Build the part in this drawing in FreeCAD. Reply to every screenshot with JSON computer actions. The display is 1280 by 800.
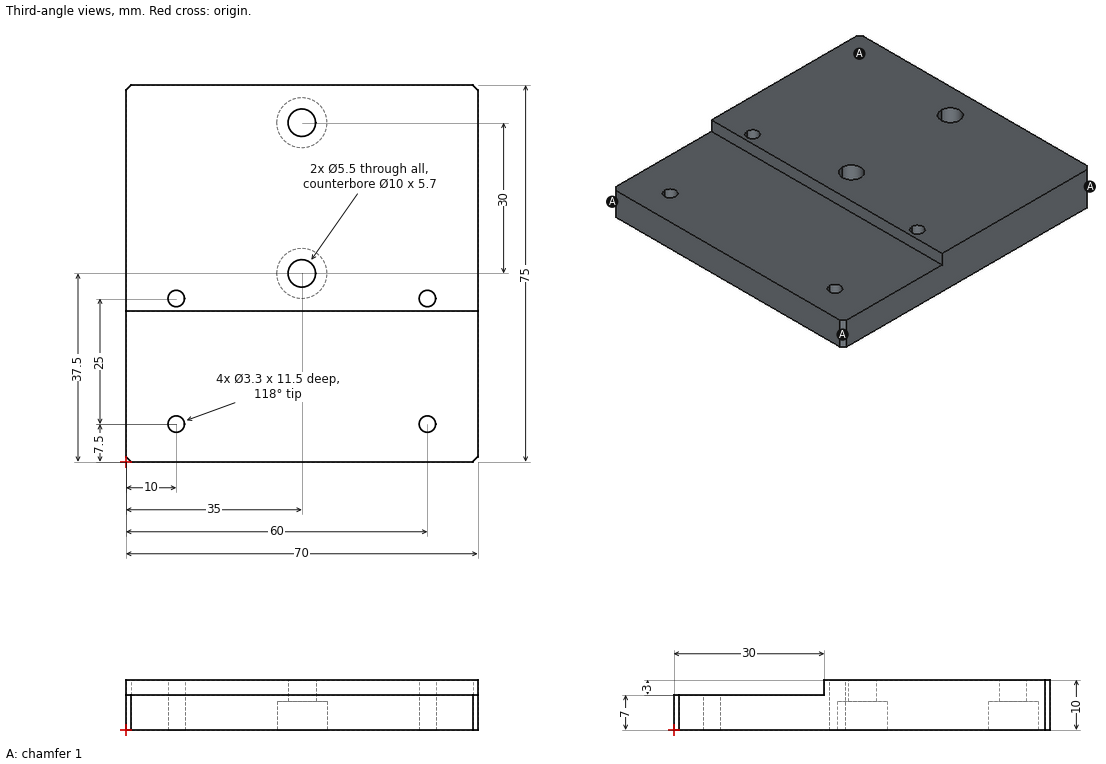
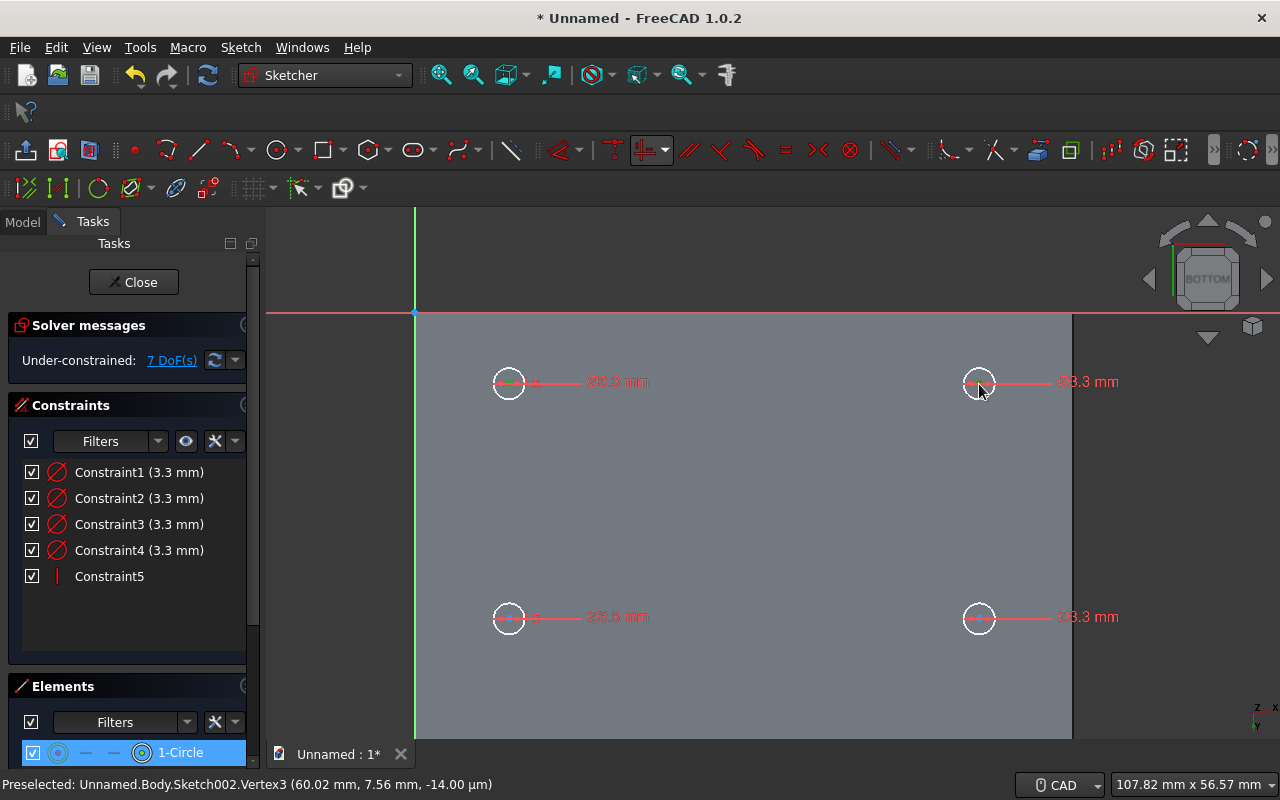
{"action": "key", "text": "h"}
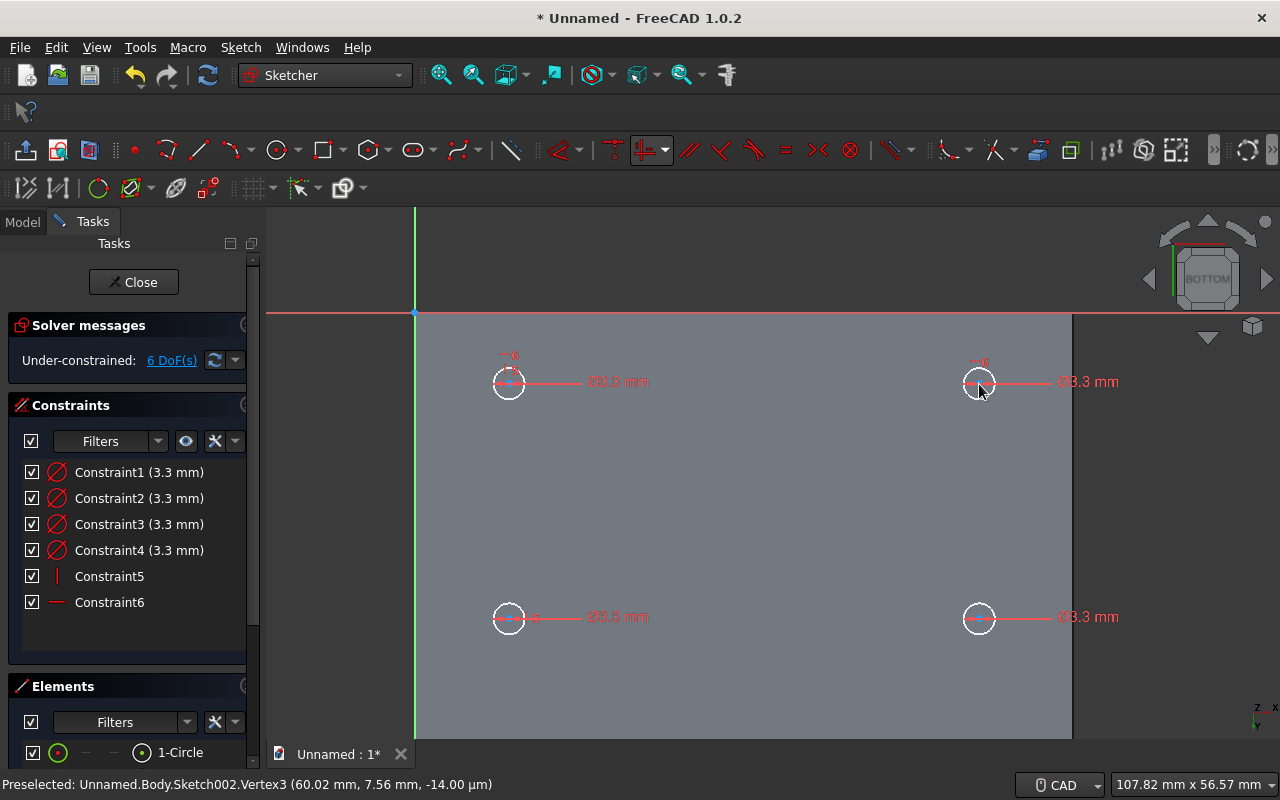
{"action": "left_click", "coordinate": [979, 384]}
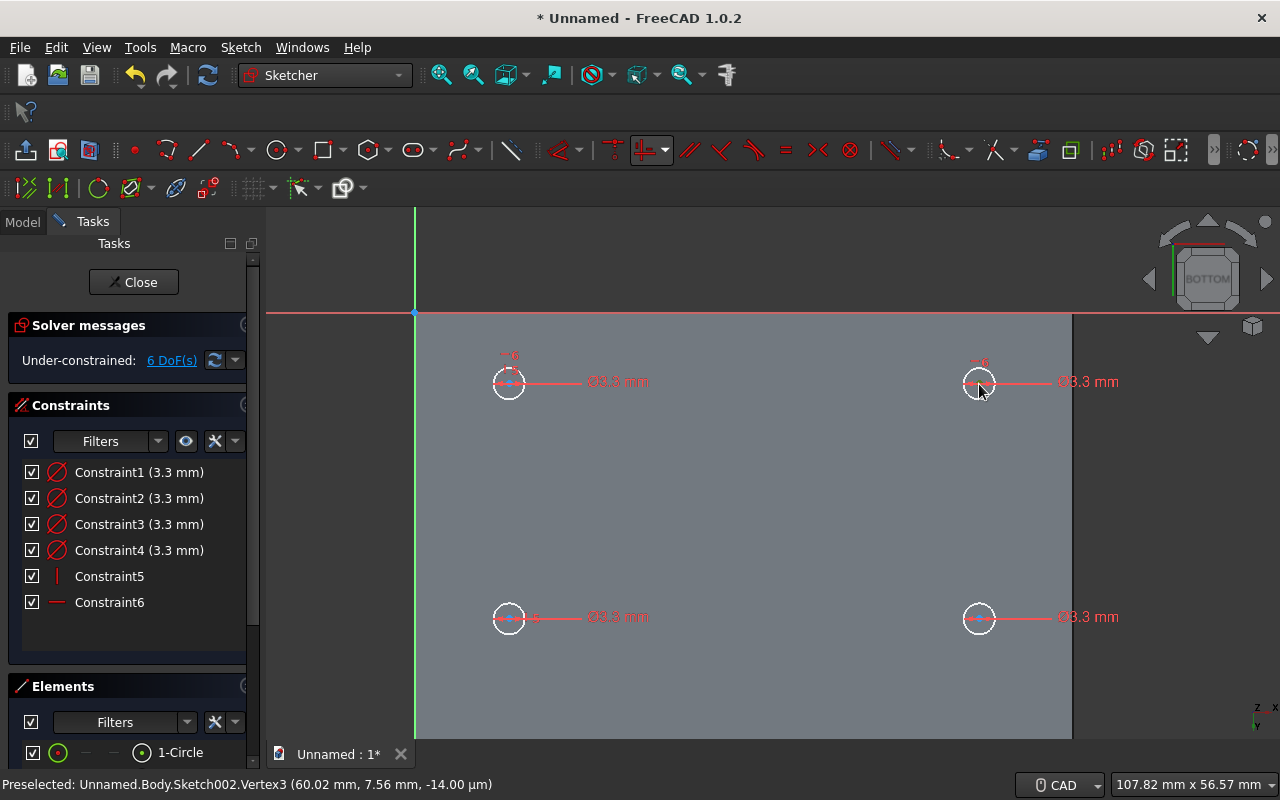
{"action": "left_click", "coordinate": [979, 619]}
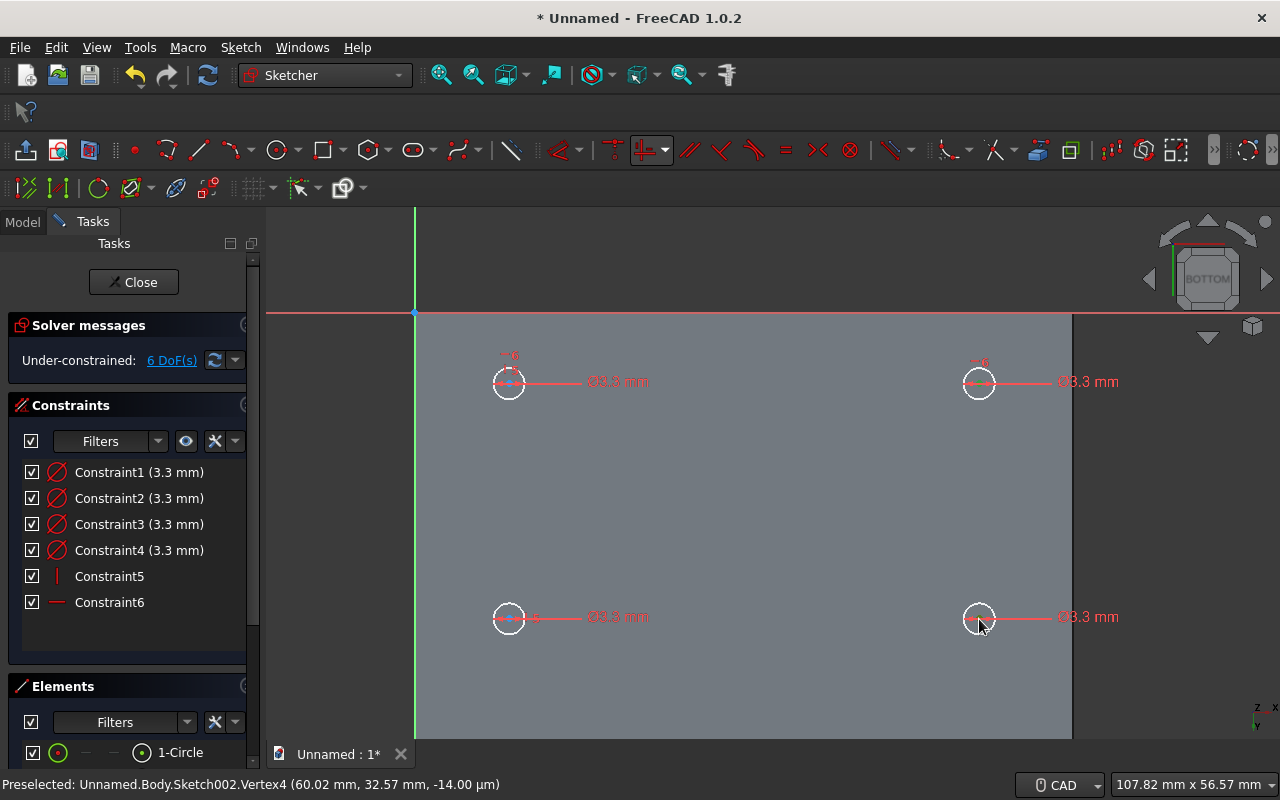
{"action": "key", "text": "v"}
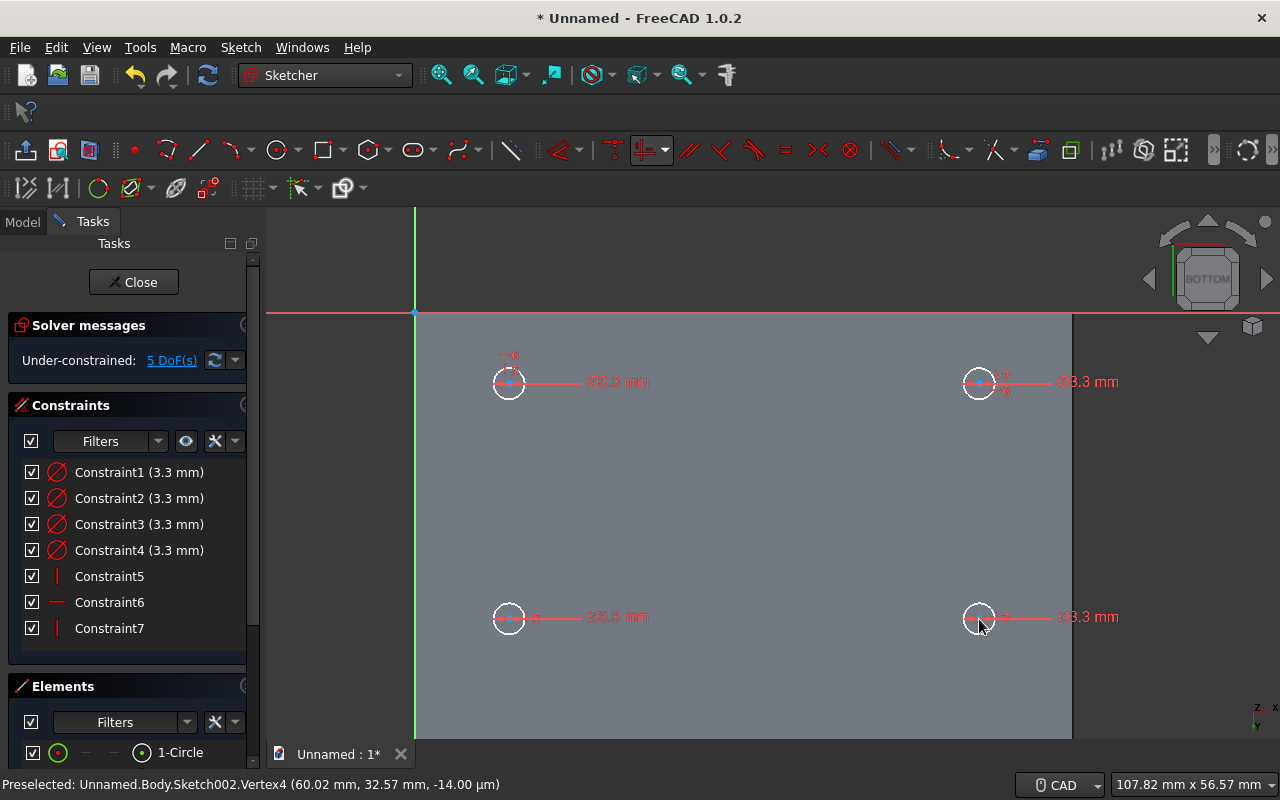
{"action": "left_click", "coordinate": [509, 619]}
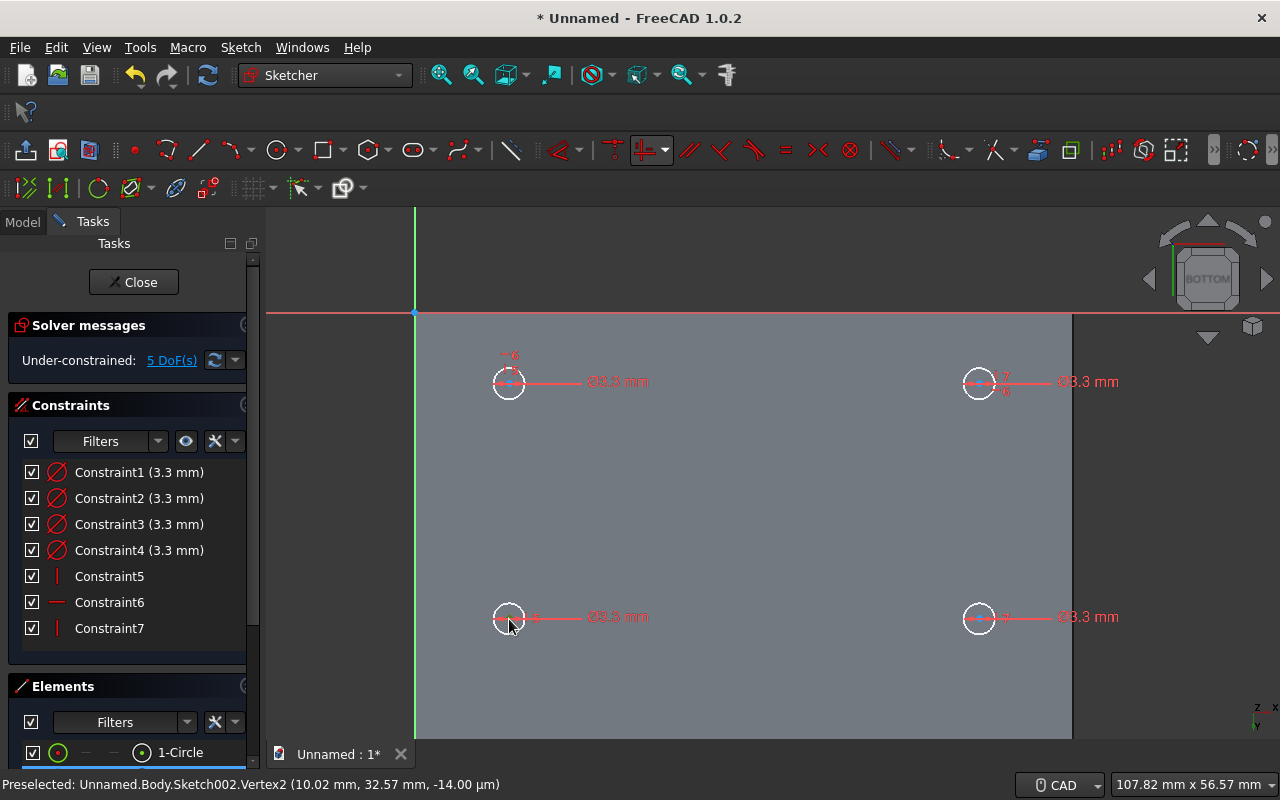
{"action": "left_click", "coordinate": [979, 619]}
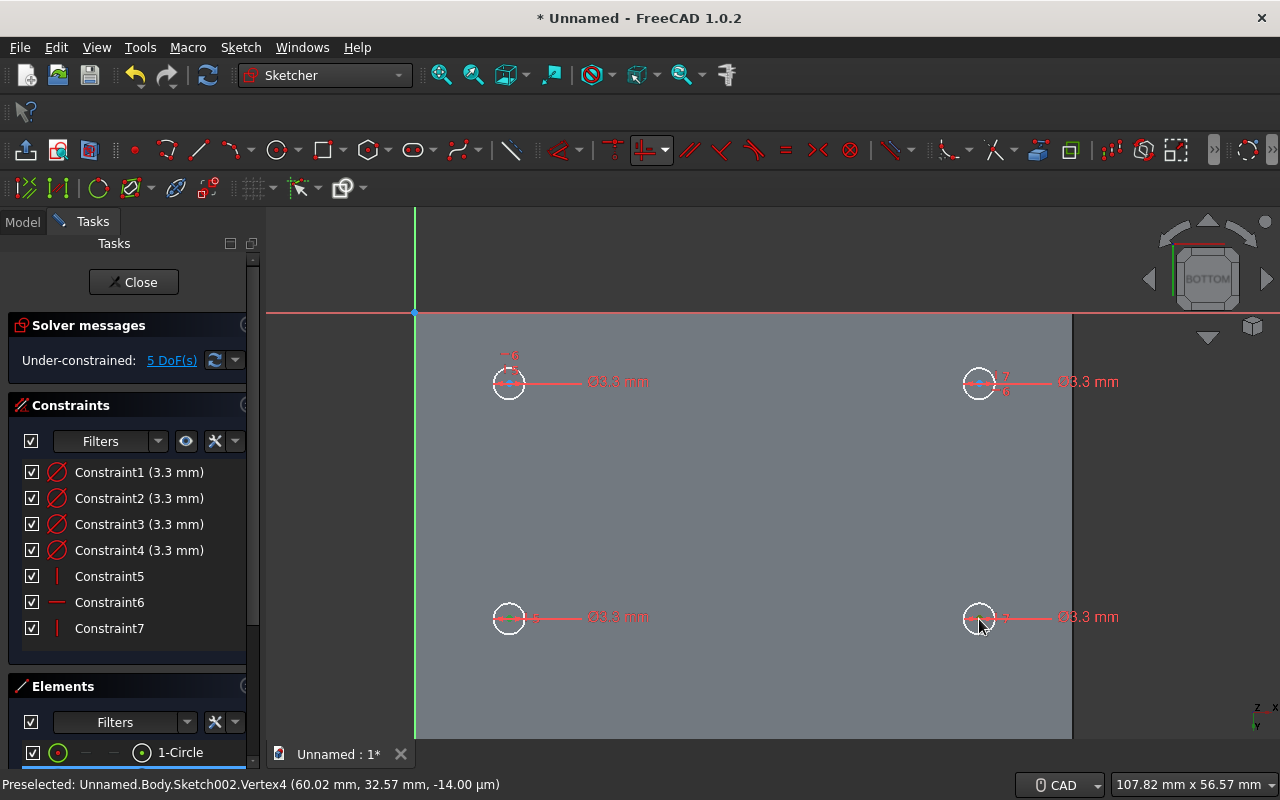
{"action": "left_click", "coordinate": [668, 150]}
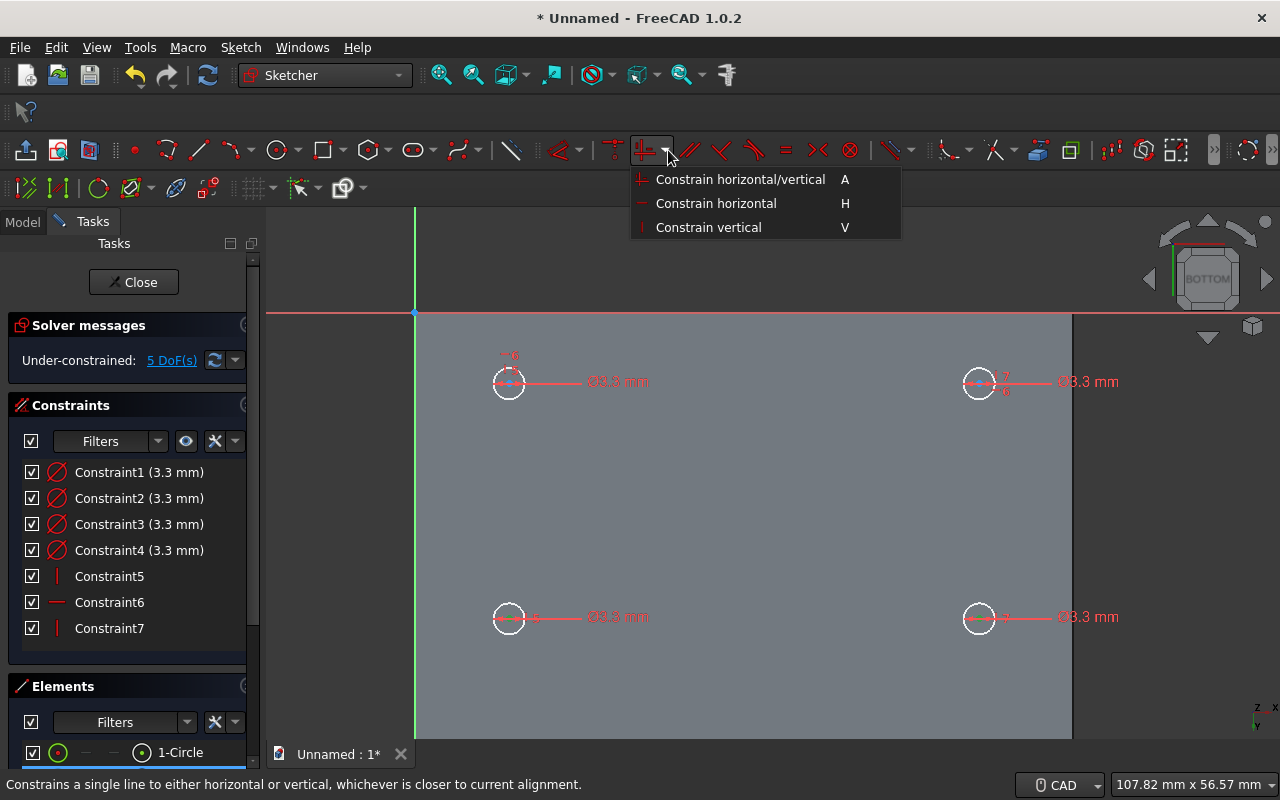
{"action": "left_click", "coordinate": [766, 203]}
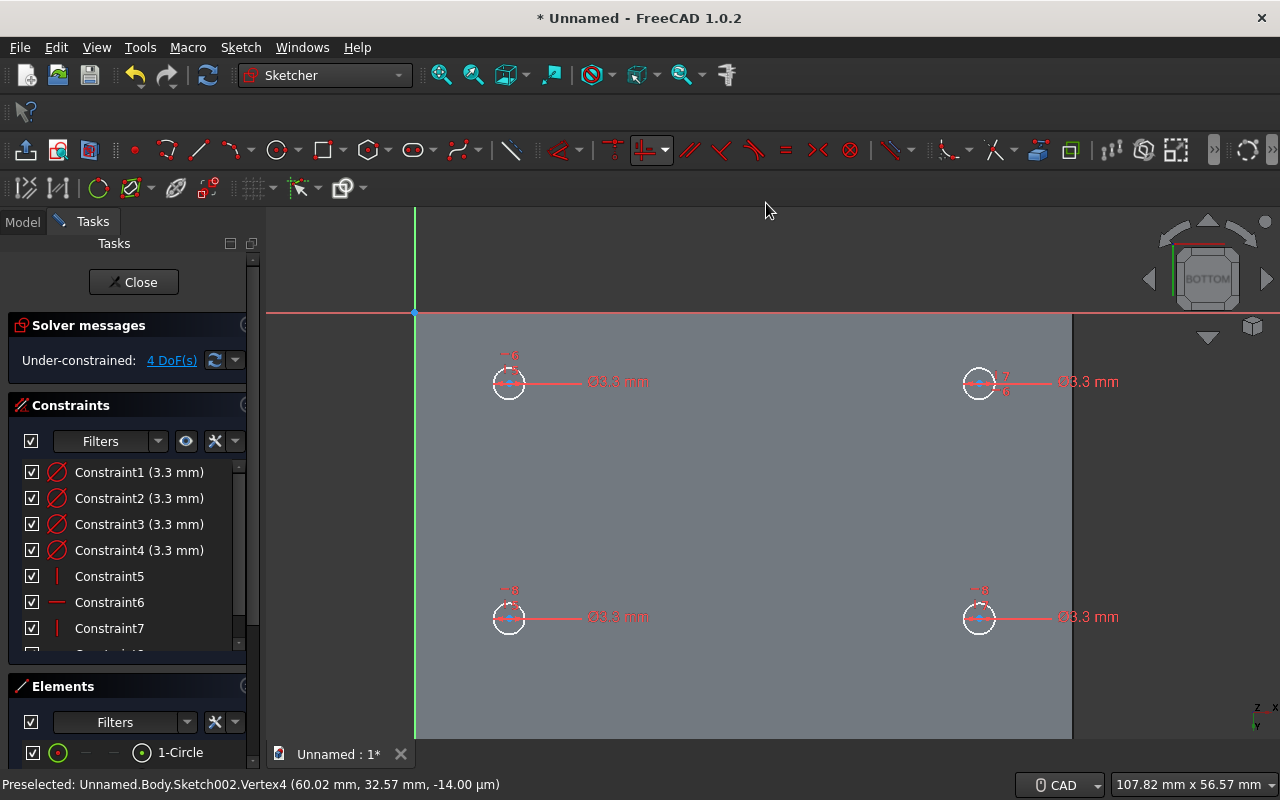
{"action": "left_click", "coordinate": [558, 150]}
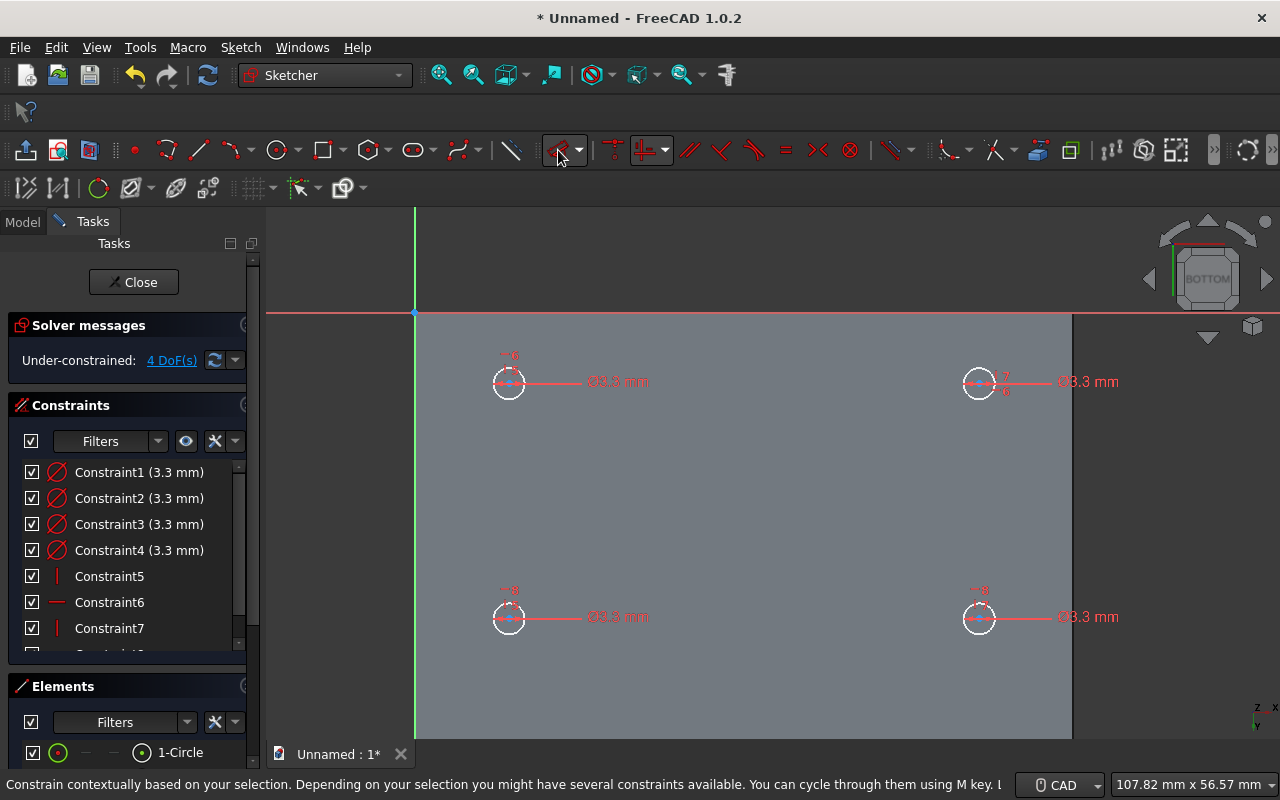
{"action": "left_click", "coordinate": [509, 384]}
{"action": "left_click", "coordinate": [462, 279]}